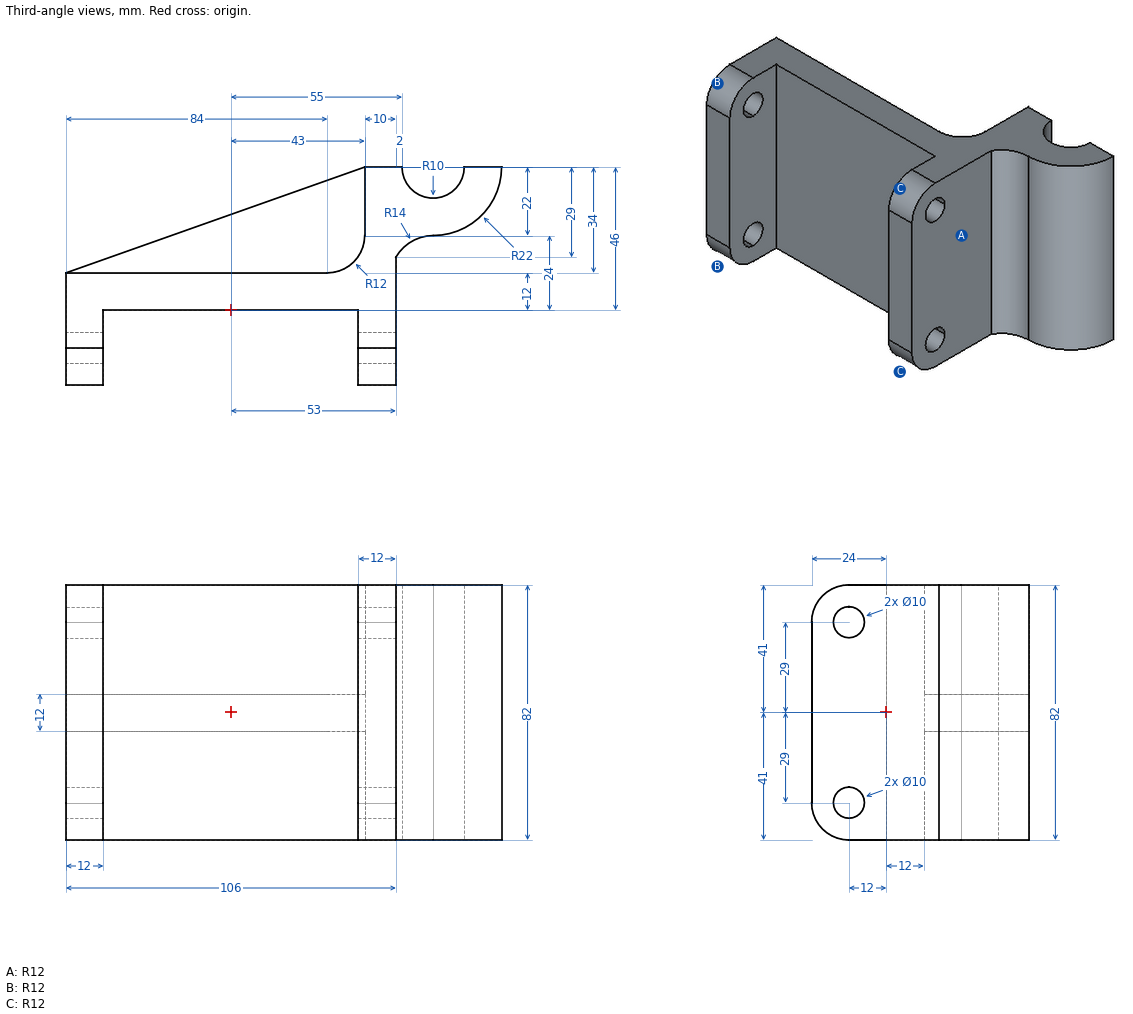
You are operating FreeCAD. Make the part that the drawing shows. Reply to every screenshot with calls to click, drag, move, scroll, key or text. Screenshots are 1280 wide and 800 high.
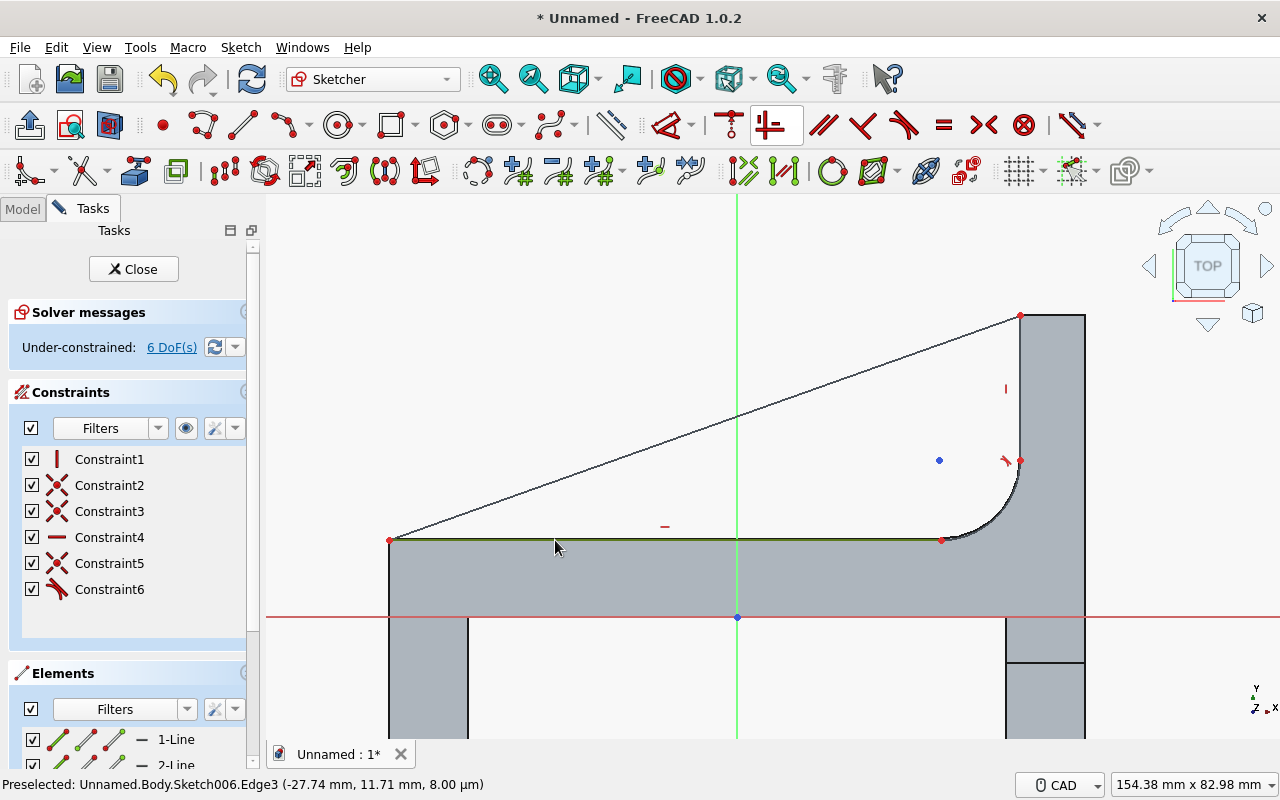
click(977, 531)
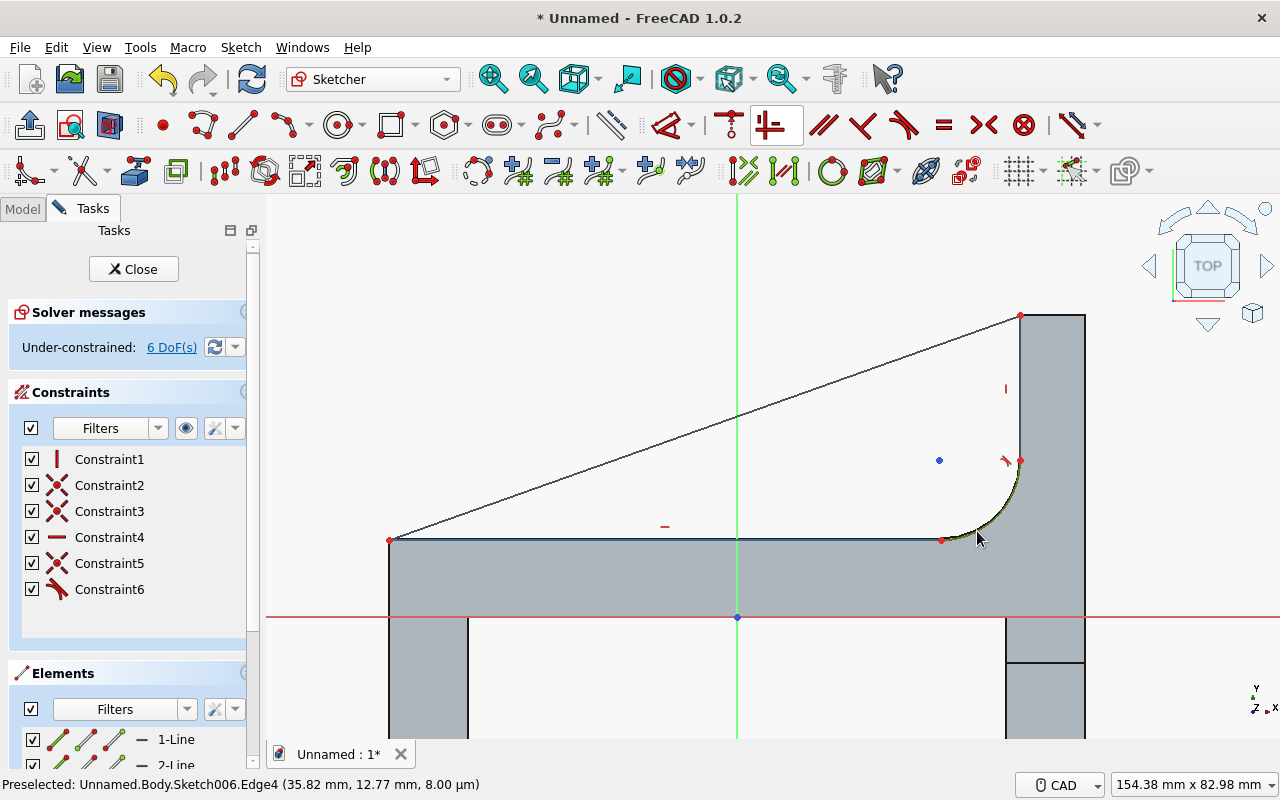
key(t)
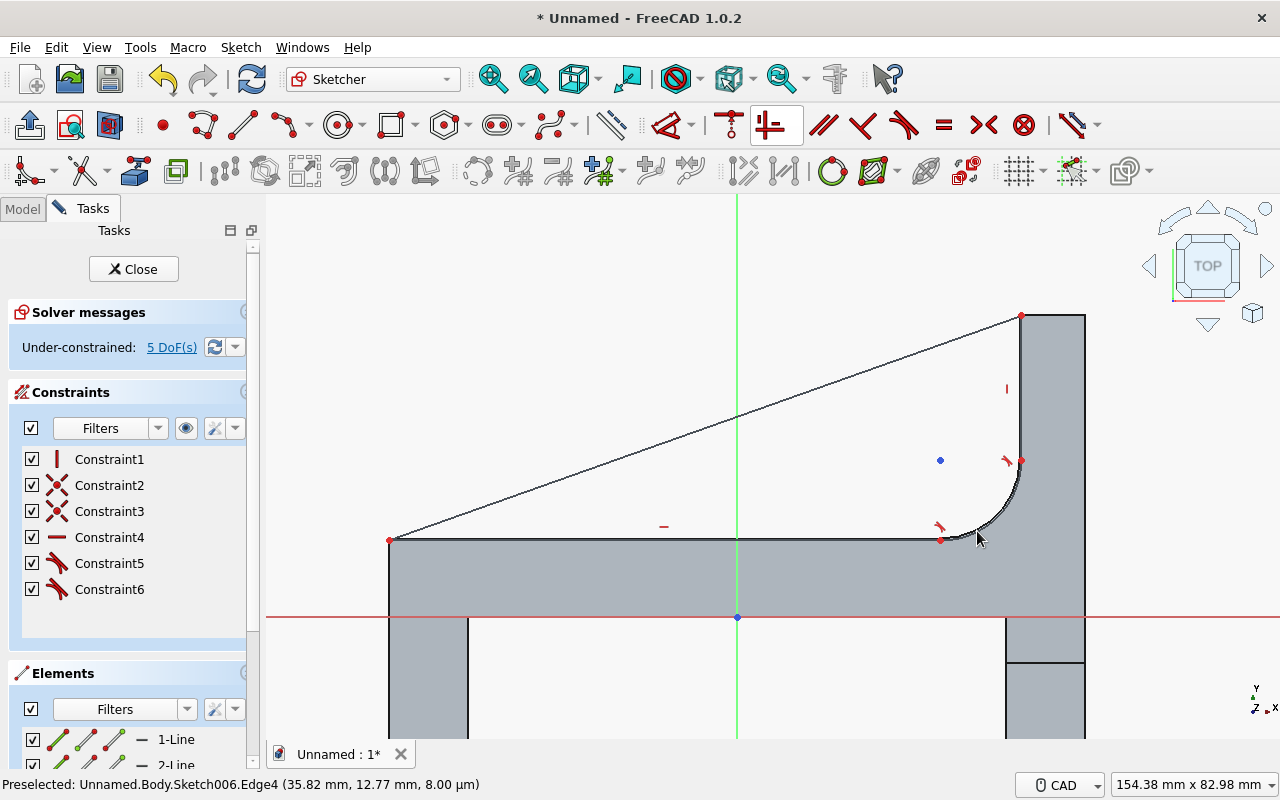
key(d)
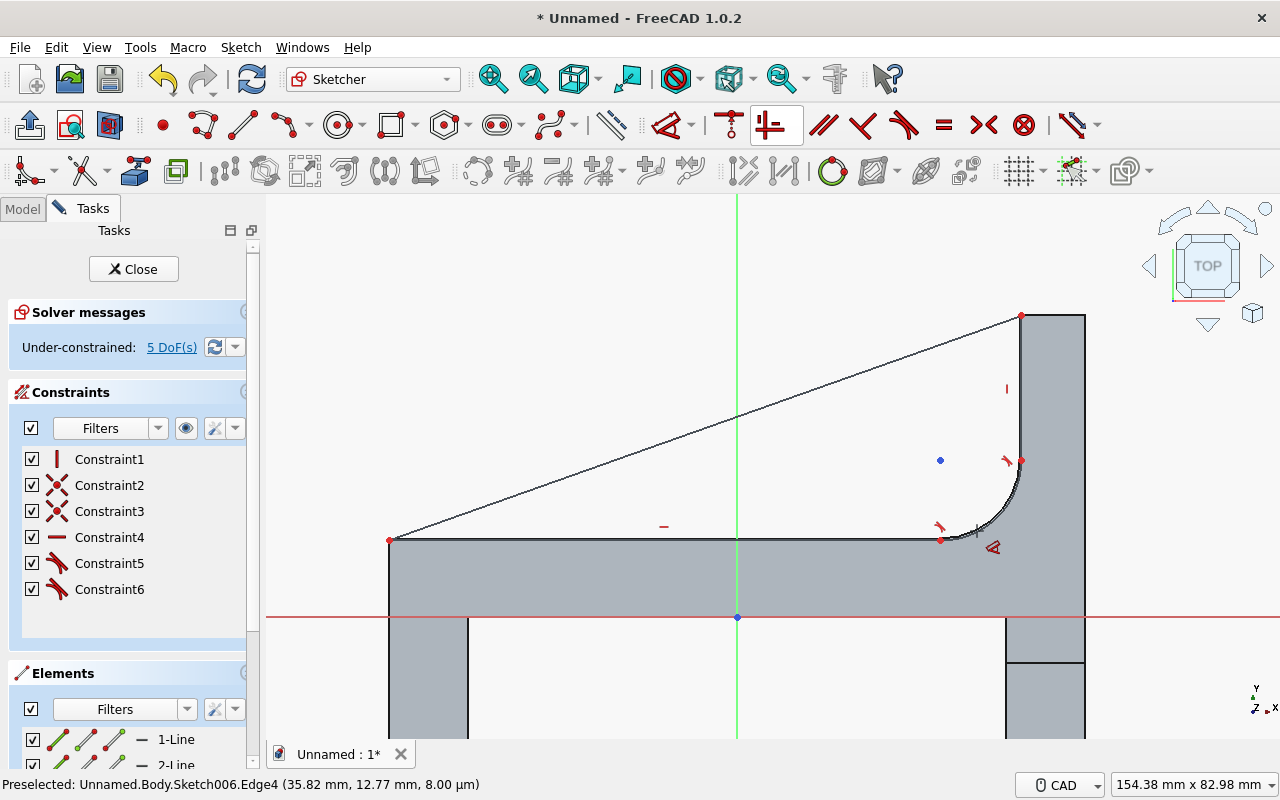
click(977, 532)
click(991, 561)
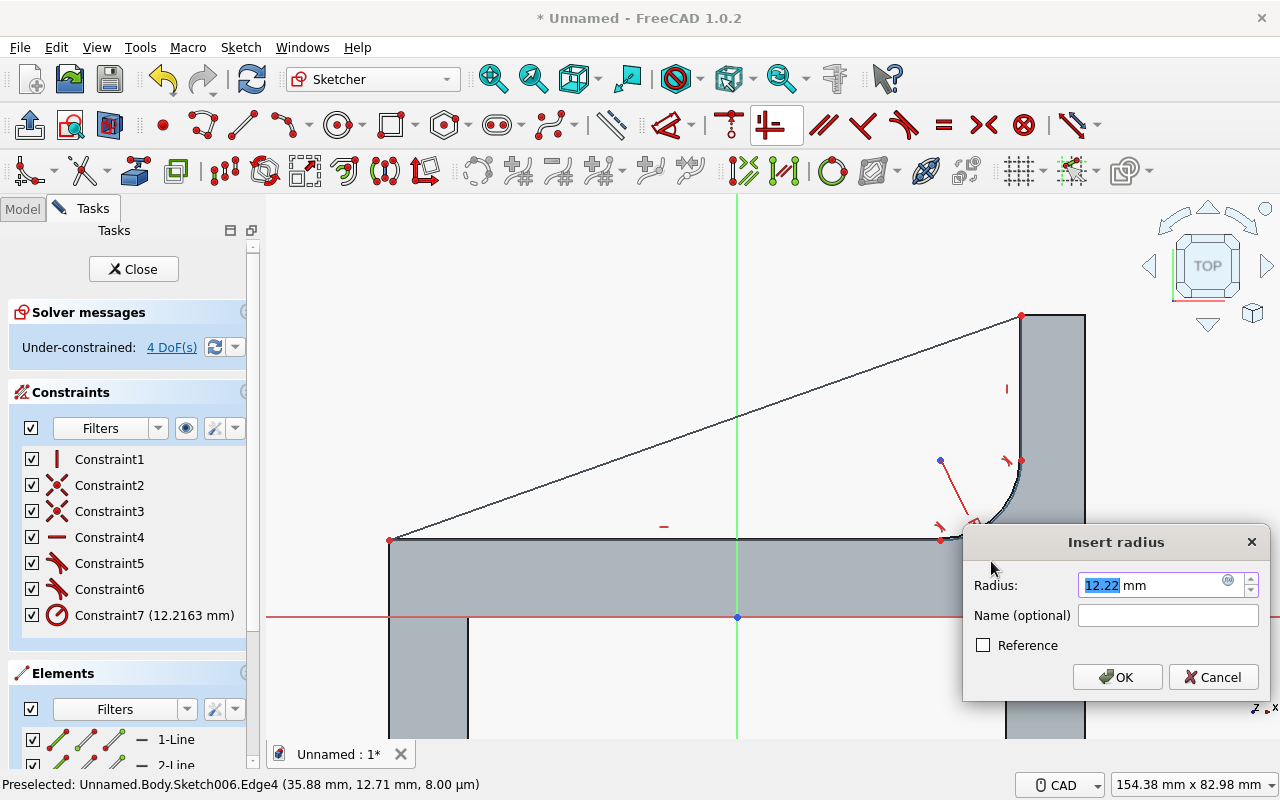
text(12)
key(Return)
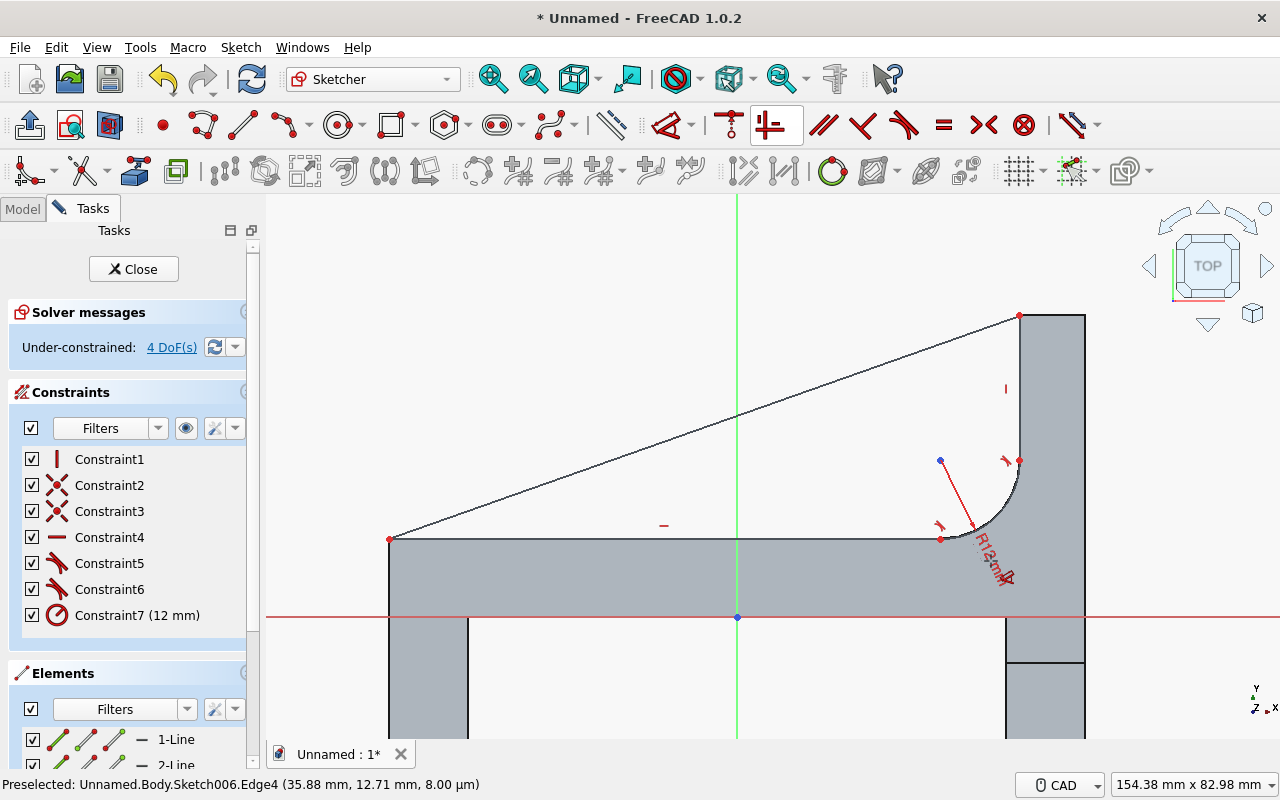
click(1020, 417)
click(1054, 388)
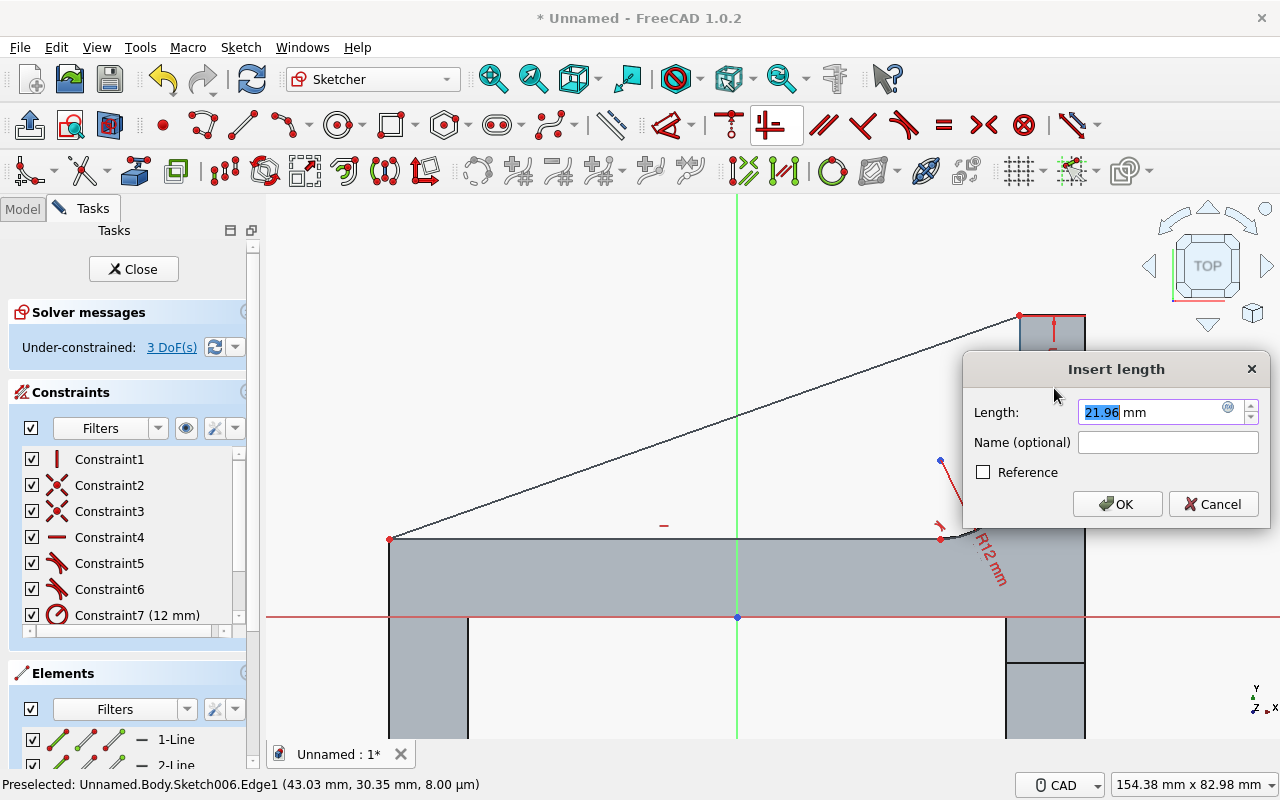
text(22)
key(Return)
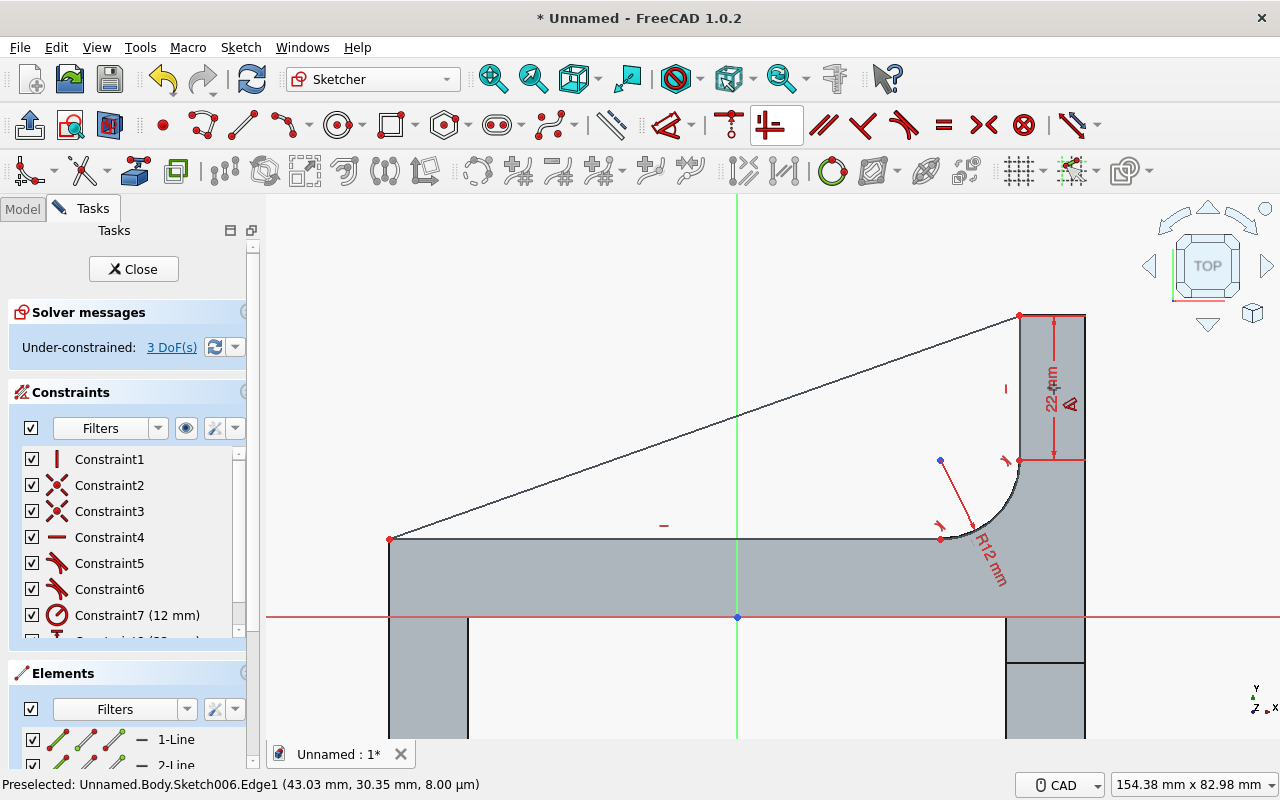
click(555, 539)
click(665, 573)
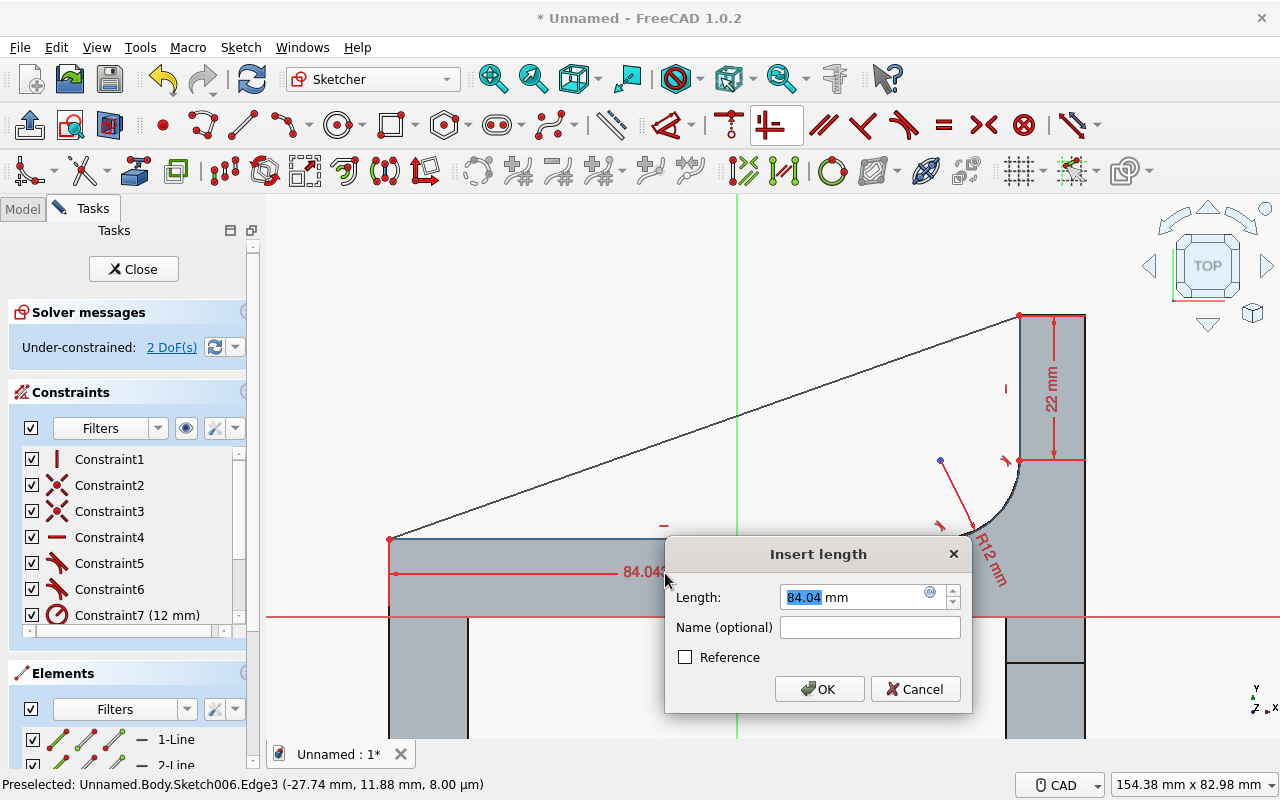
text(84)
key(Return)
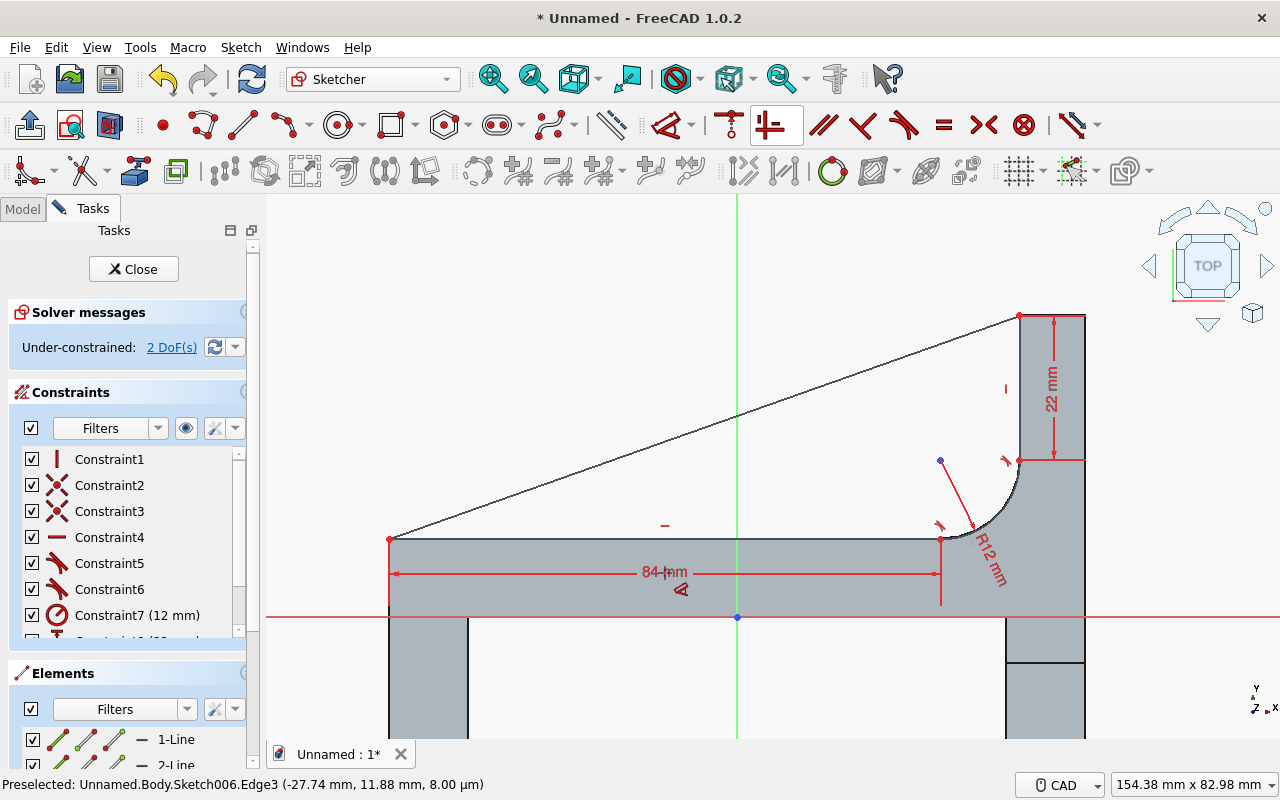
click(1020, 460)
click(879, 651)